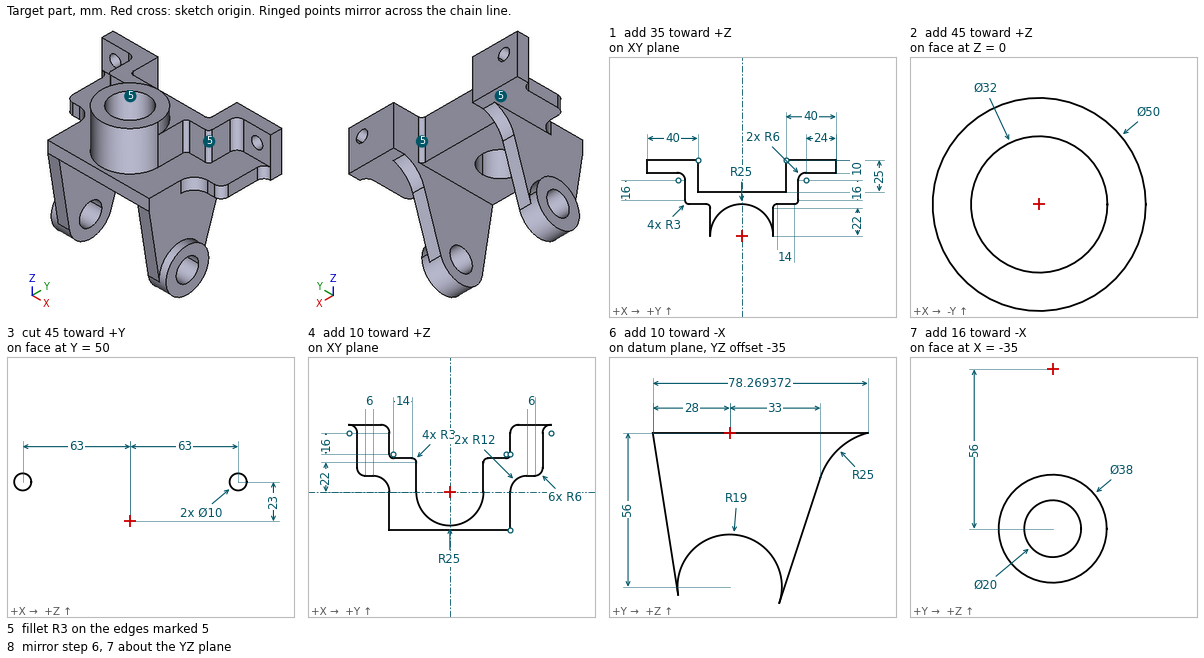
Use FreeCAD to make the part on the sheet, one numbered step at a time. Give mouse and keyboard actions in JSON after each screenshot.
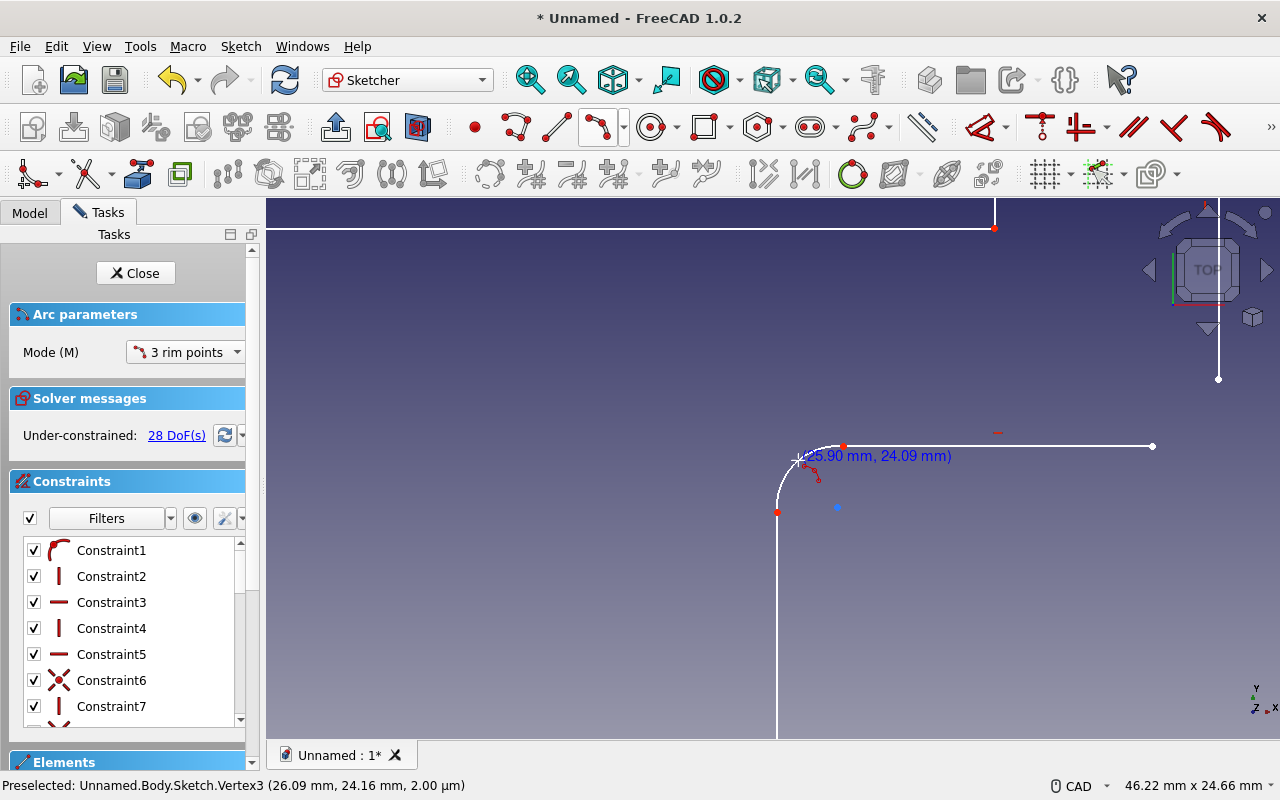
{"action": "scroll", "coordinate": [798, 496], "scroll_direction": "down", "scroll_amount": 9}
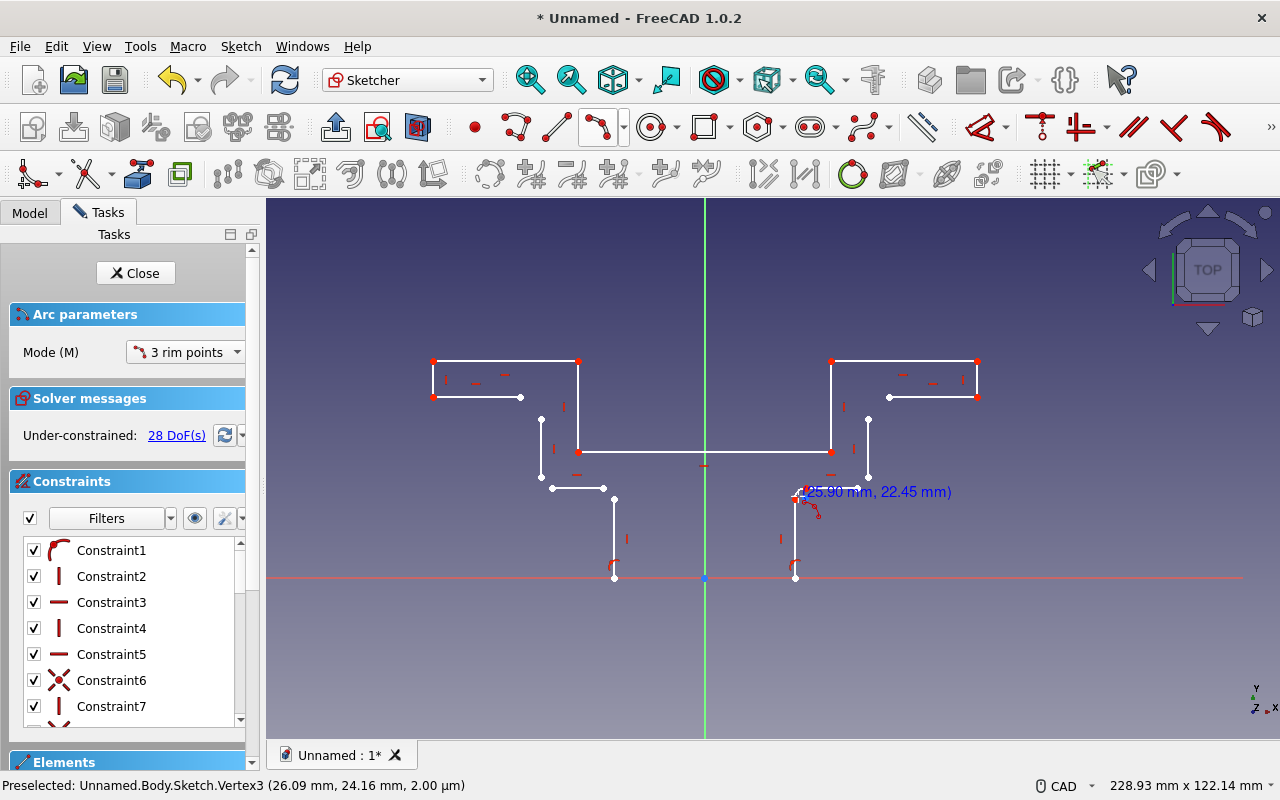
{"action": "left_click", "coordinate": [857, 488]}
{"action": "left_click", "coordinate": [868, 477]}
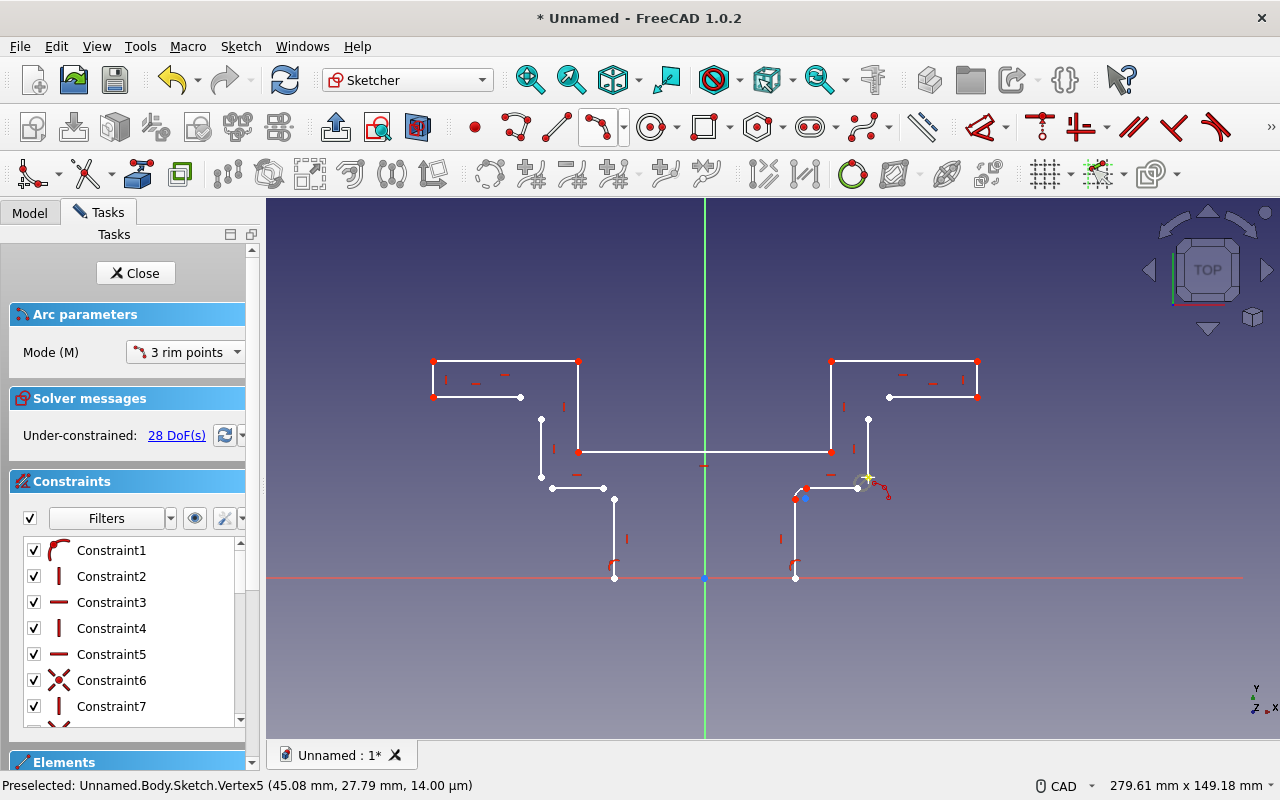
{"action": "scroll", "coordinate": [865, 484], "scroll_direction": "up", "scroll_amount": 9}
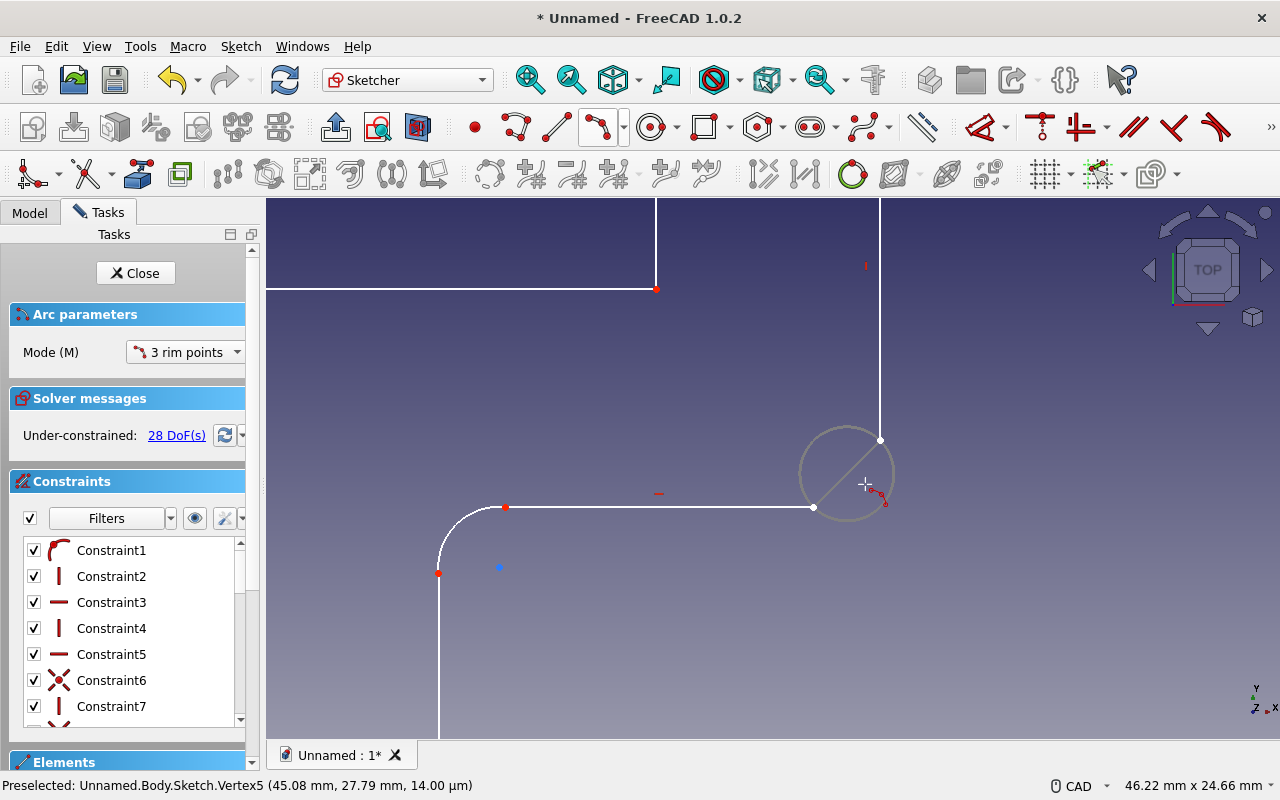
{"action": "left_click", "coordinate": [859, 482]}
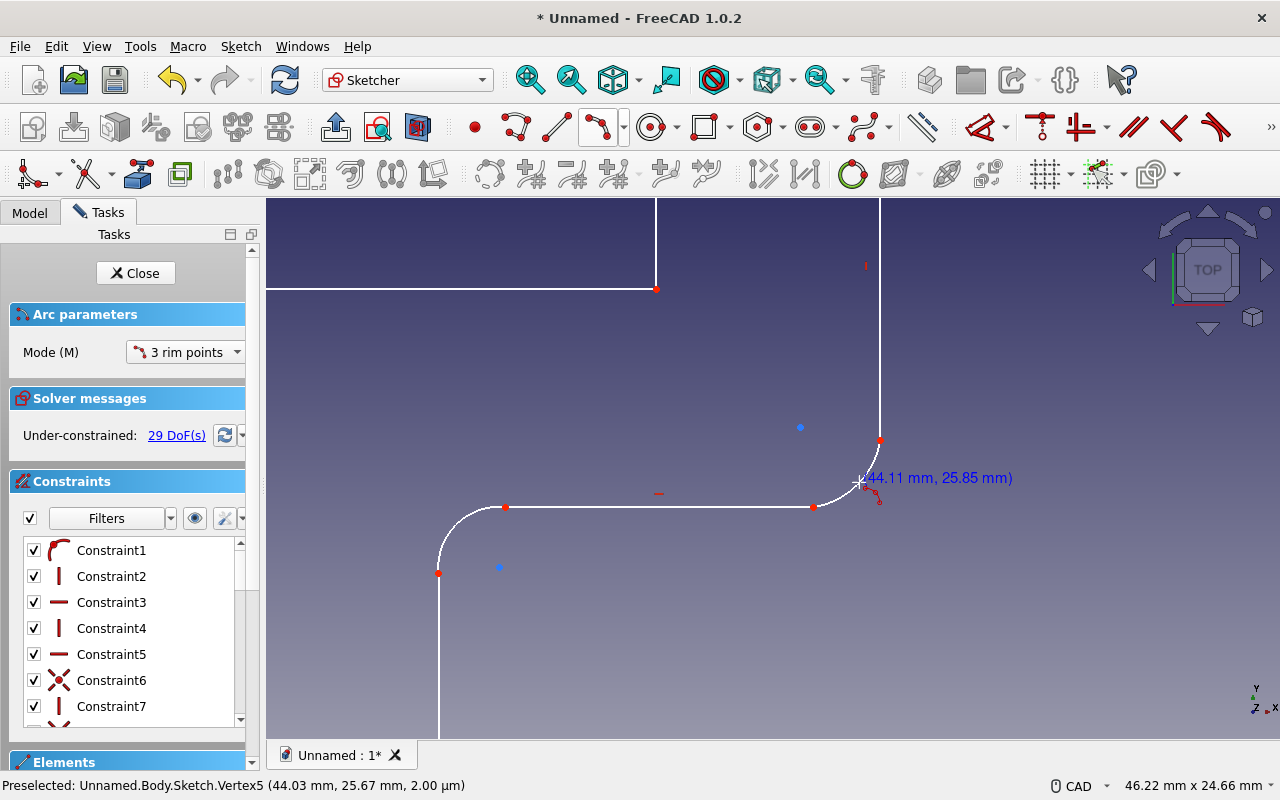
{"action": "scroll", "coordinate": [866, 484], "scroll_direction": "down", "scroll_amount": 9}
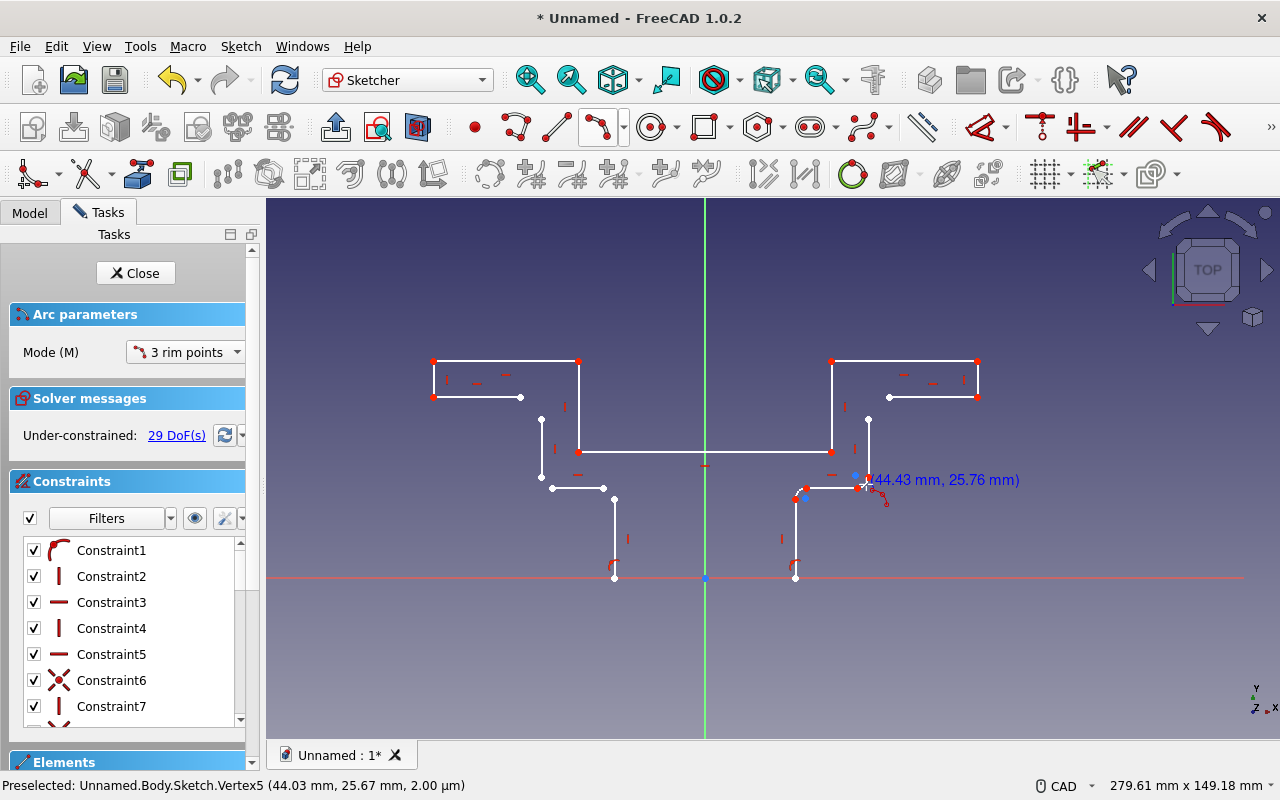
{"action": "left_click", "coordinate": [869, 419]}
{"action": "left_click", "coordinate": [890, 397]}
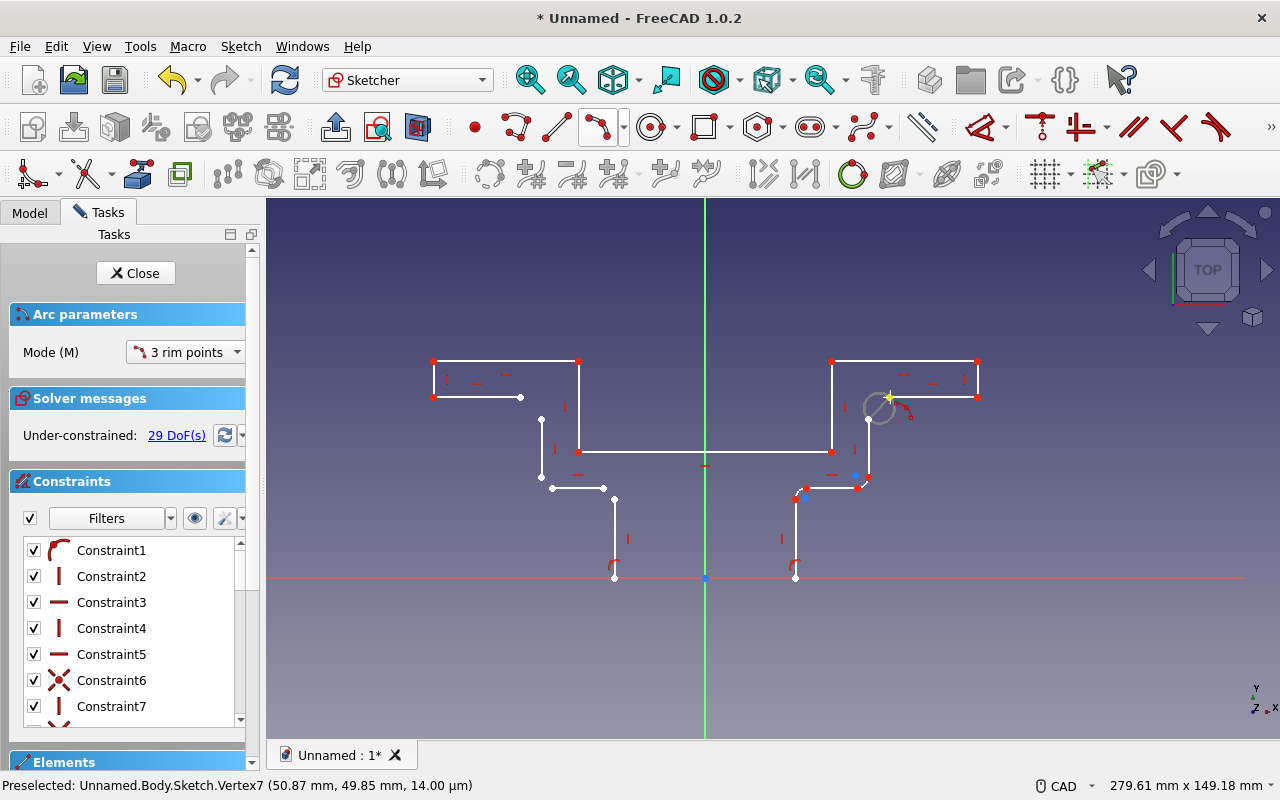
{"action": "scroll", "coordinate": [875, 403], "scroll_direction": "up", "scroll_amount": 5}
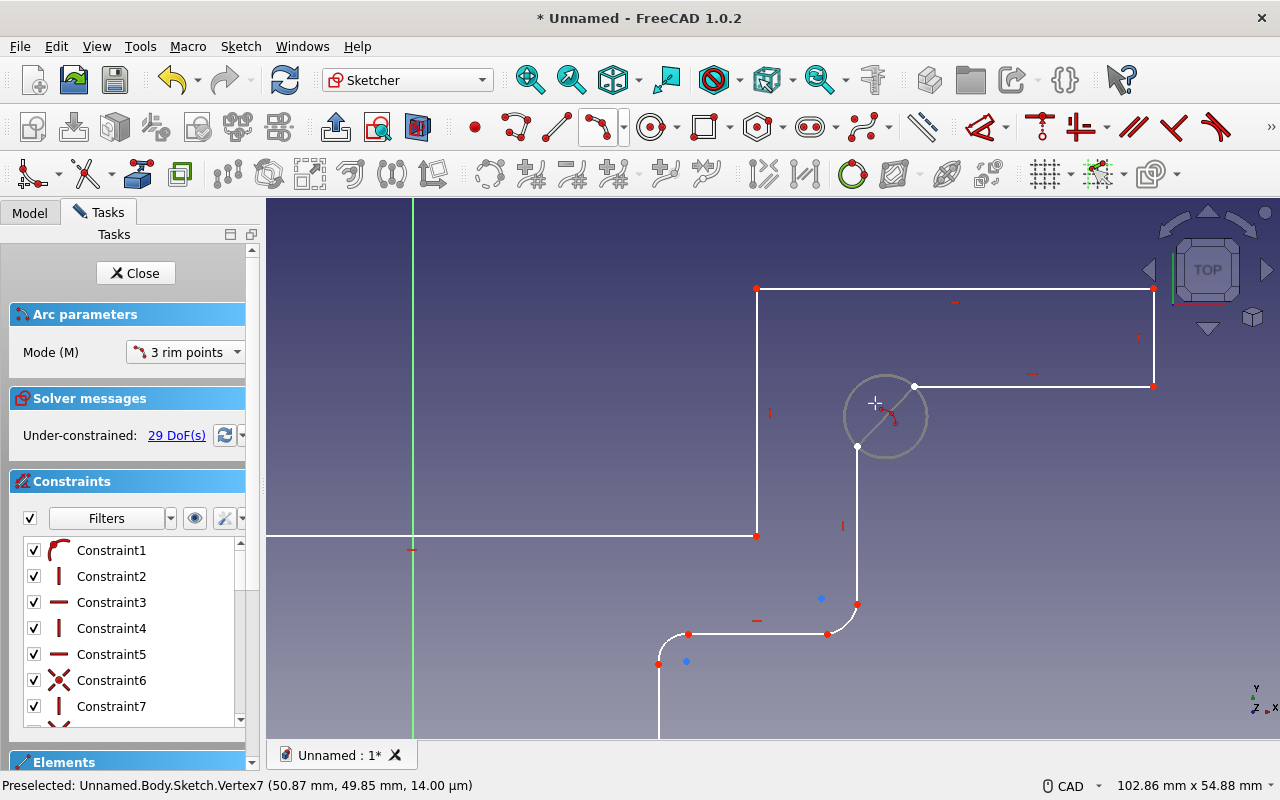
{"action": "left_click", "coordinate": [874, 403]}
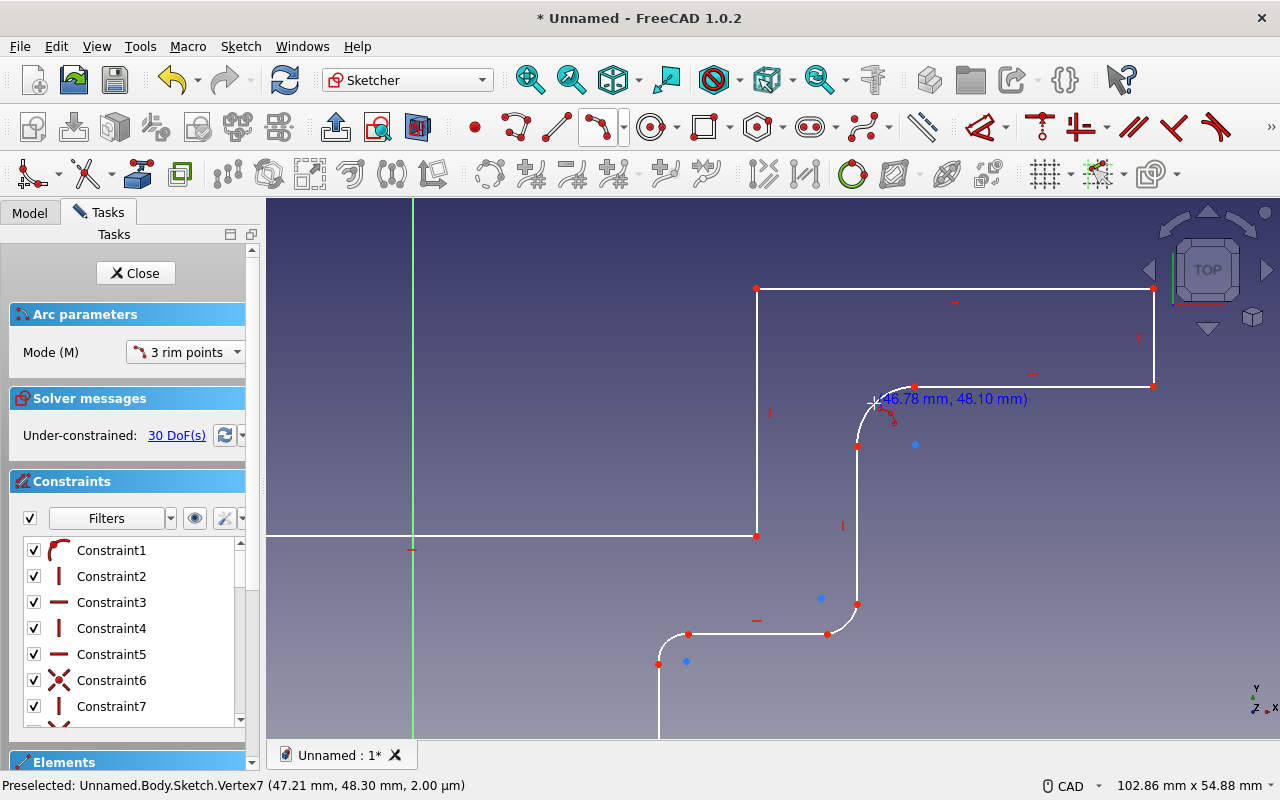
{"action": "scroll", "coordinate": [874, 402], "scroll_direction": "down", "scroll_amount": 5}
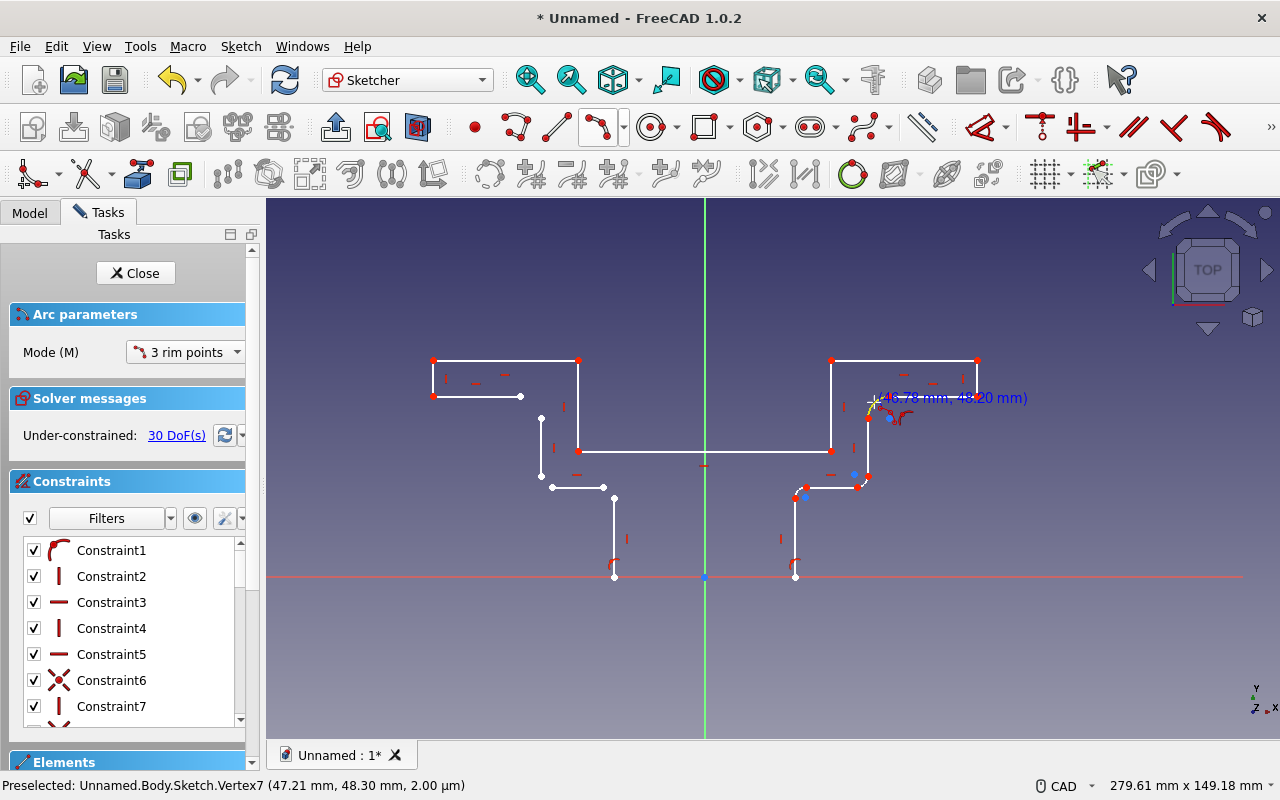
{"action": "left_click", "coordinate": [520, 397]}
{"action": "left_click", "coordinate": [541, 419]}